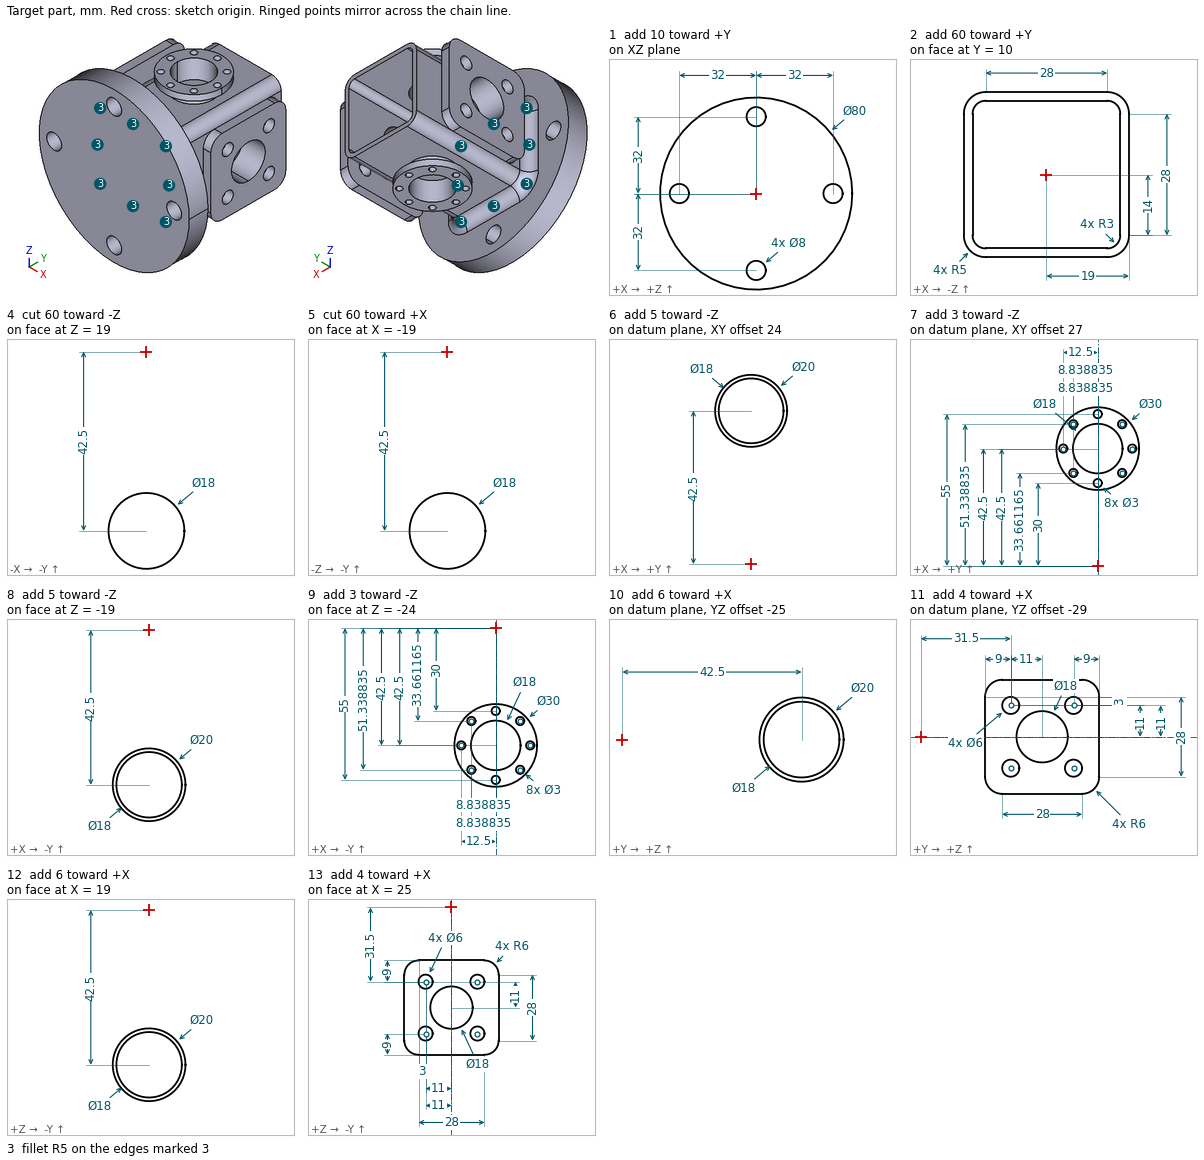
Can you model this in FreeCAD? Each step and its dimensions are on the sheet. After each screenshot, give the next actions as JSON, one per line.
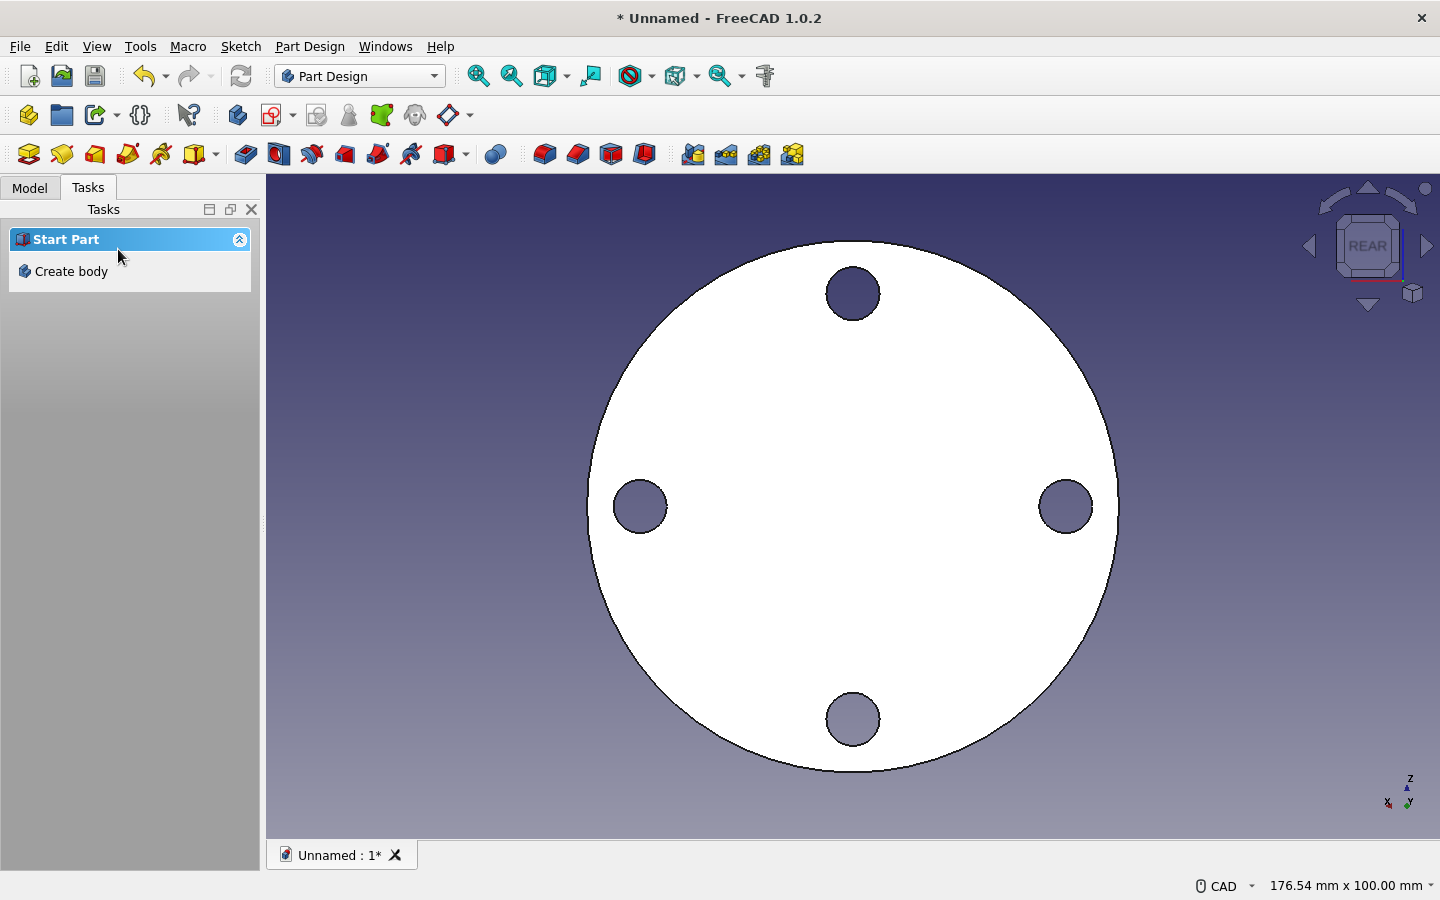
{"action": "left_click", "coordinate": [853, 505]}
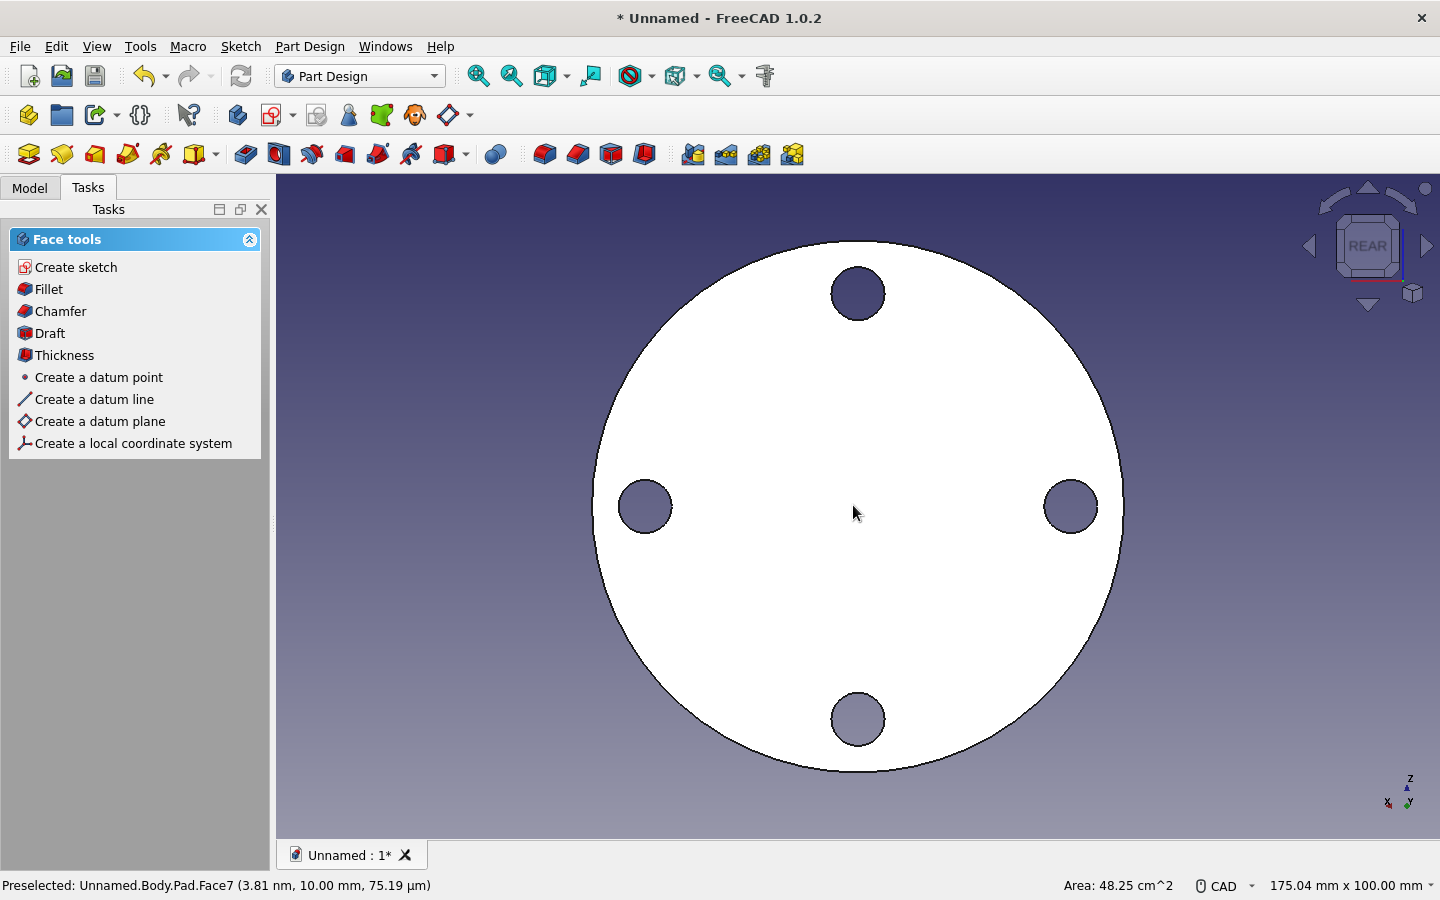
{"action": "left_click", "coordinate": [270, 116]}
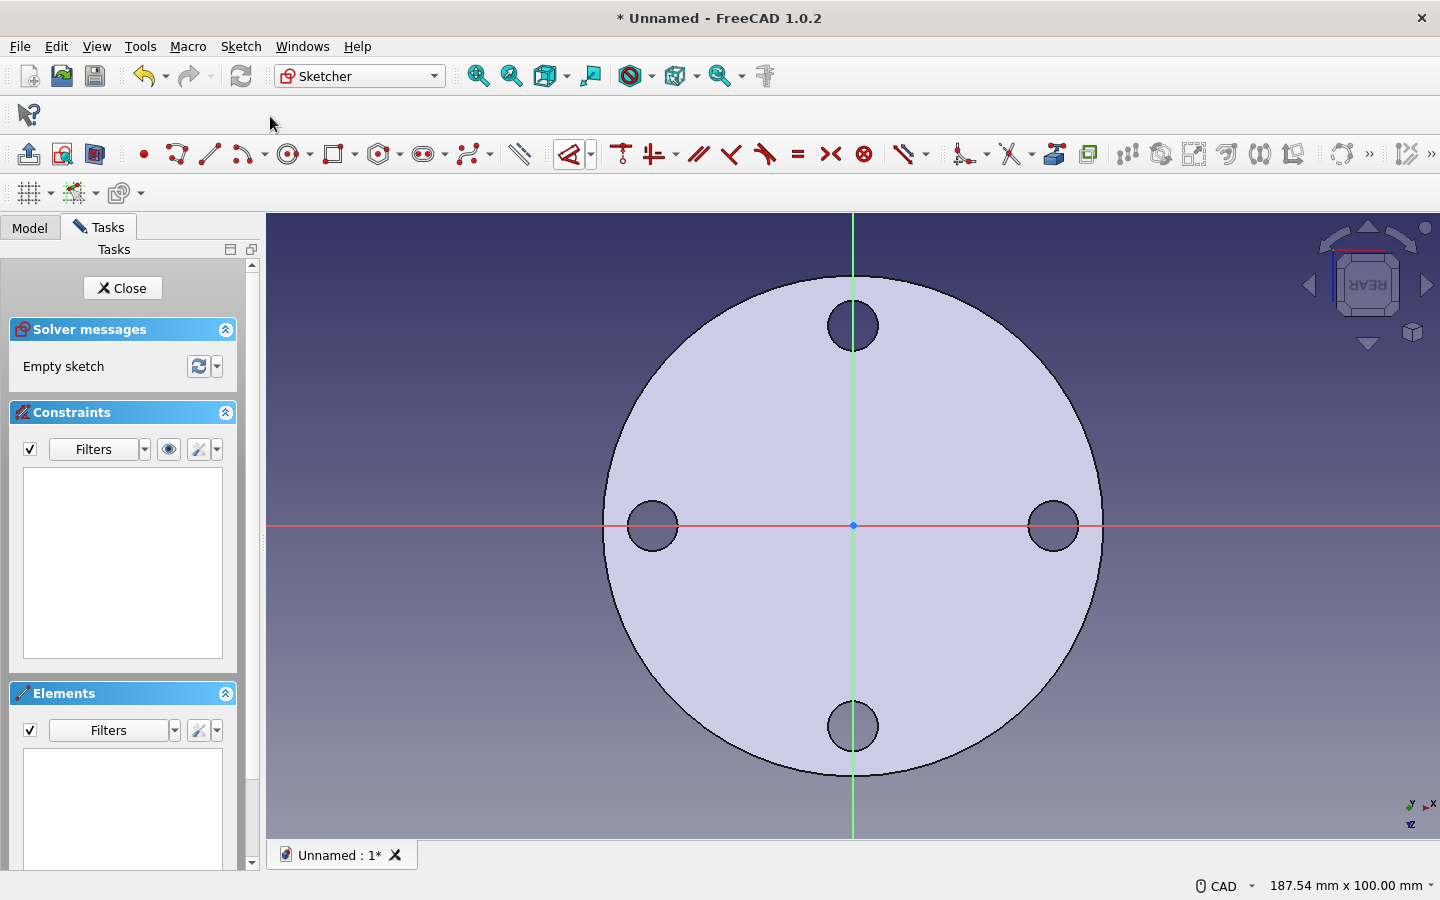
{"action": "scroll", "coordinate": [936, 526], "scroll_direction": "up", "scroll_amount": 3}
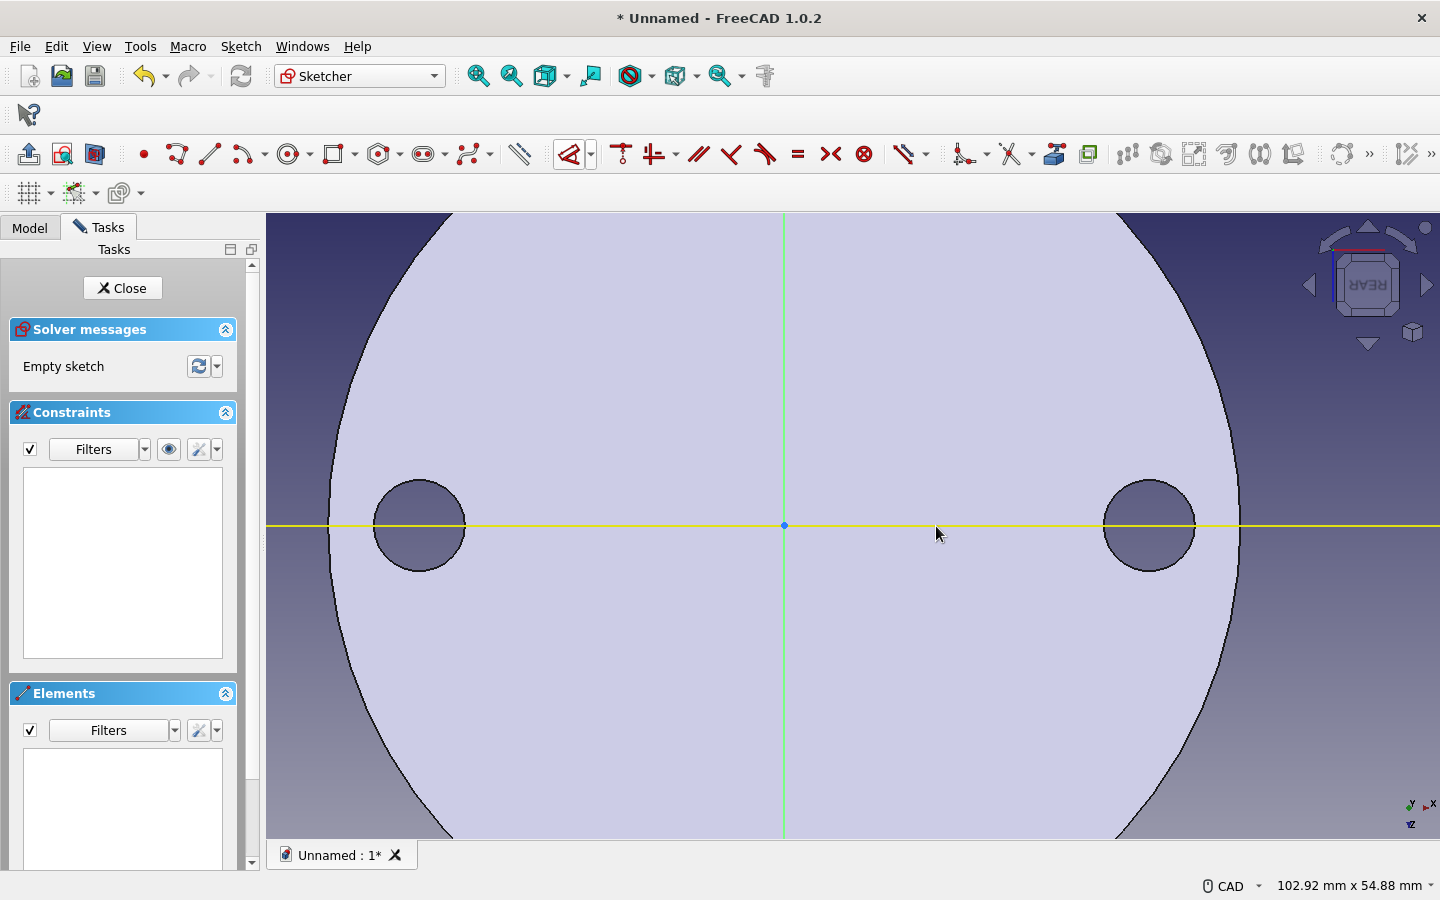
{"action": "left_click", "coordinate": [210, 154]}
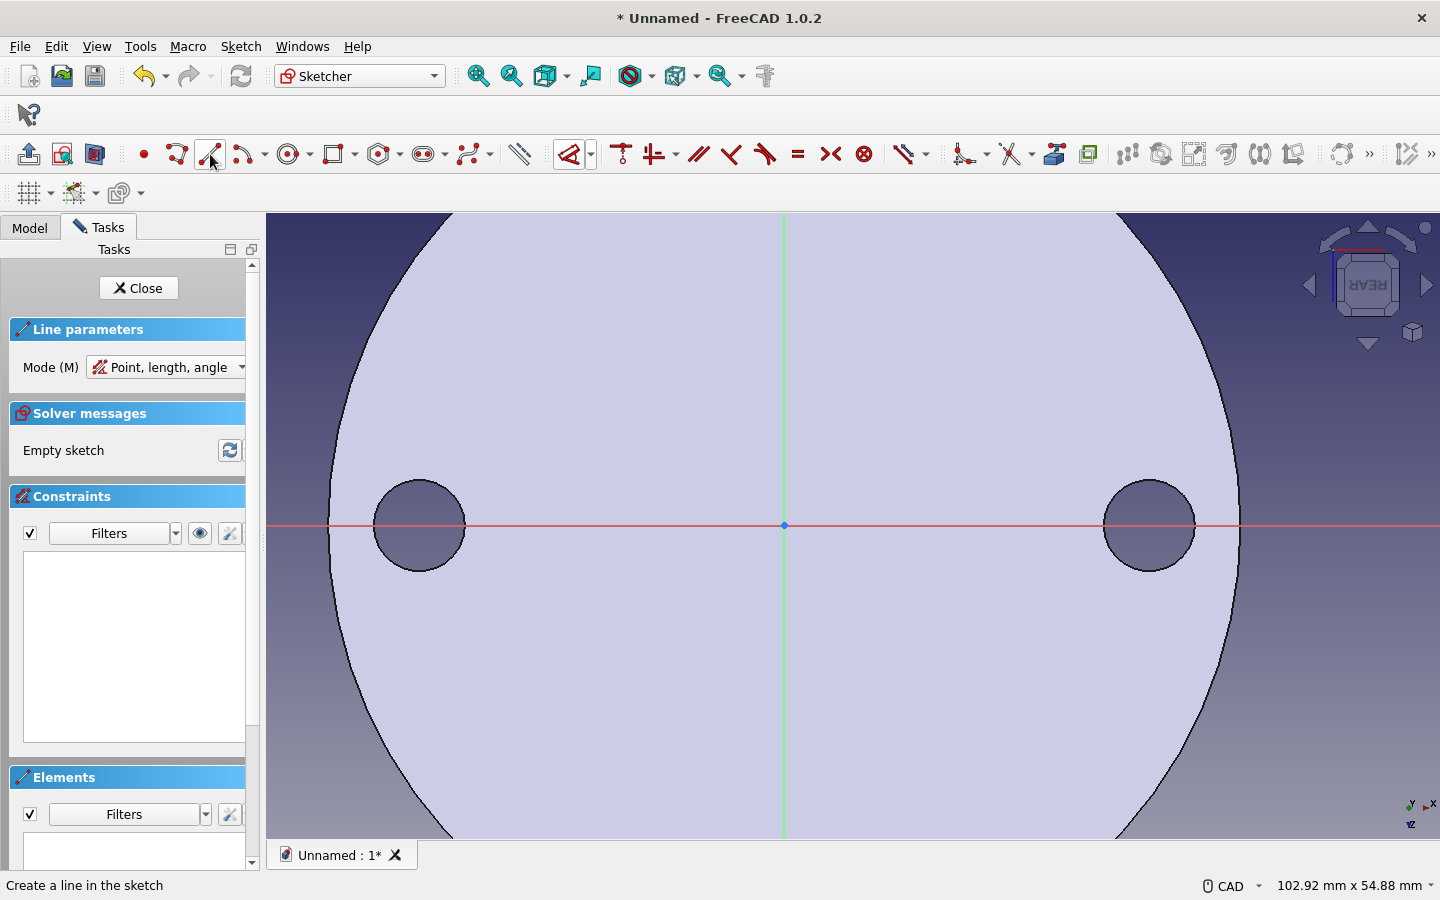
{"action": "left_click", "coordinate": [1001, 685]}
{"action": "left_click", "coordinate": [1001, 366]}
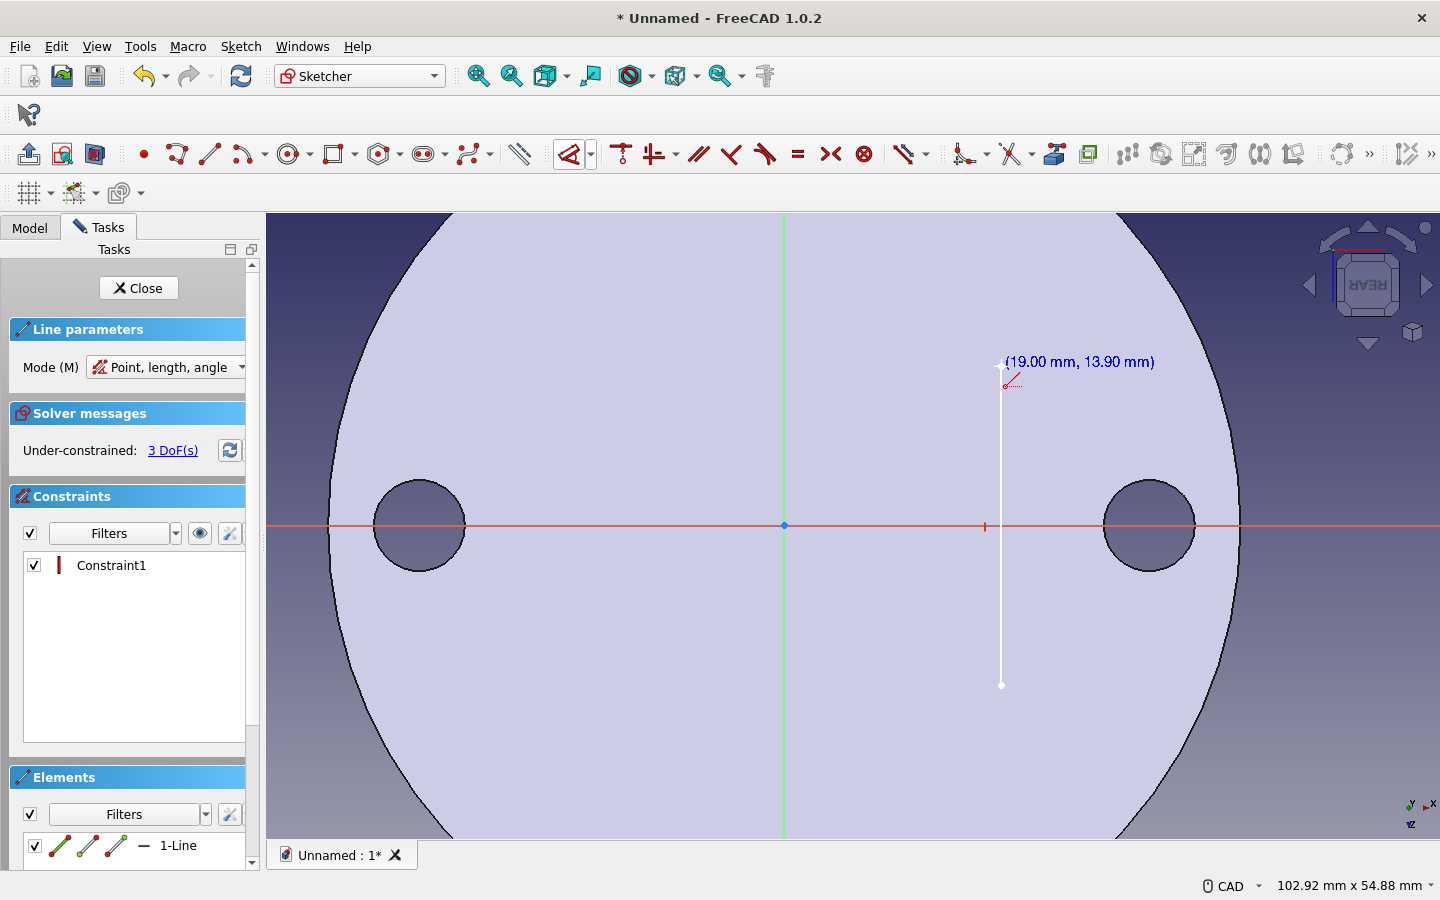
{"action": "left_click", "coordinate": [944, 309]}
{"action": "left_click", "coordinate": [625, 309]}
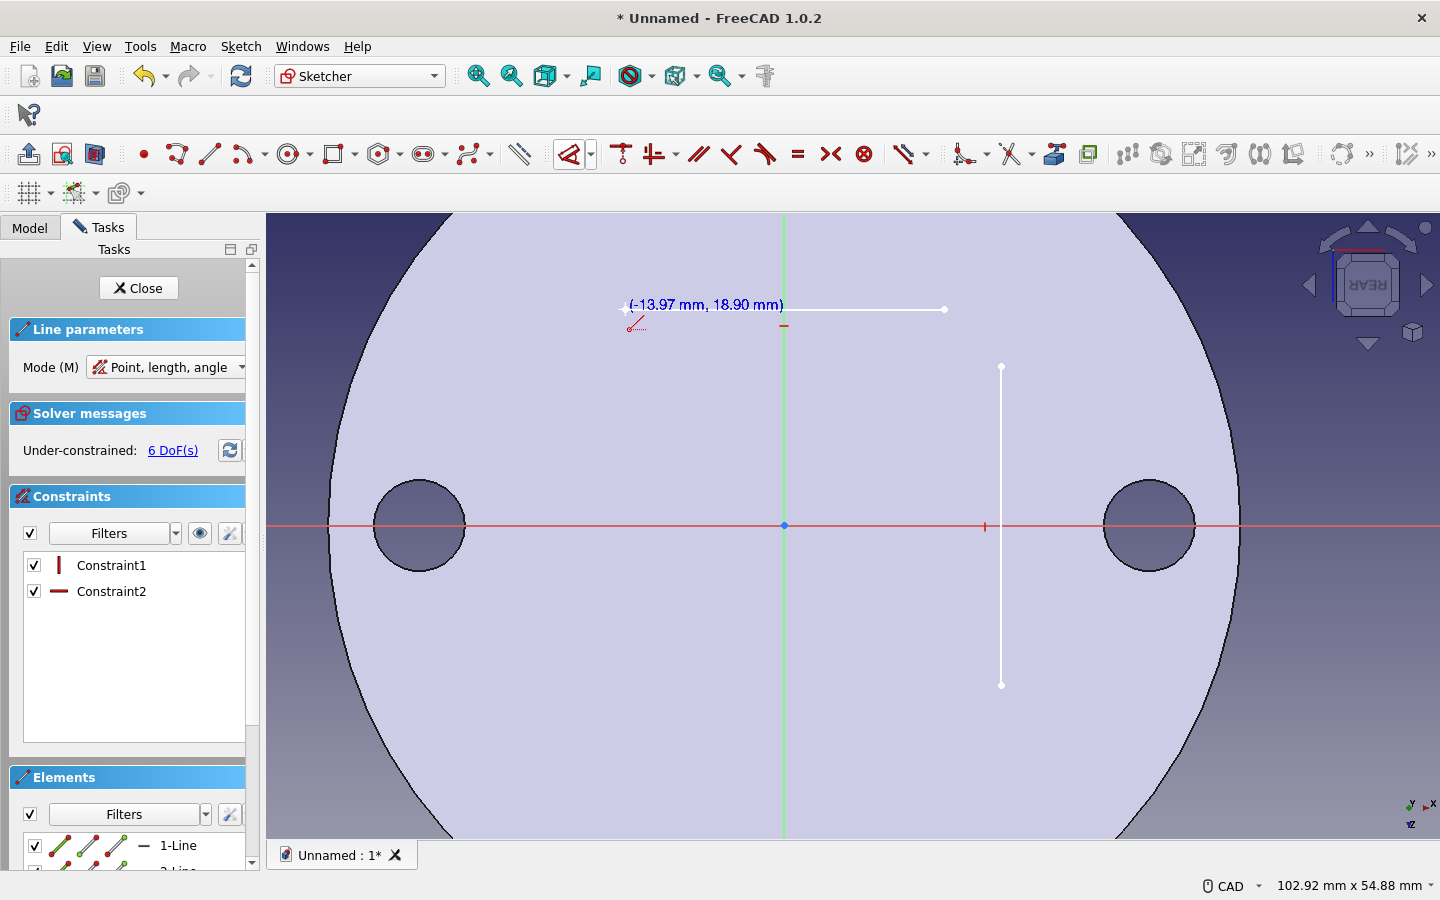
{"action": "left_click", "coordinate": [568, 366]}
{"action": "left_click", "coordinate": [568, 685]}